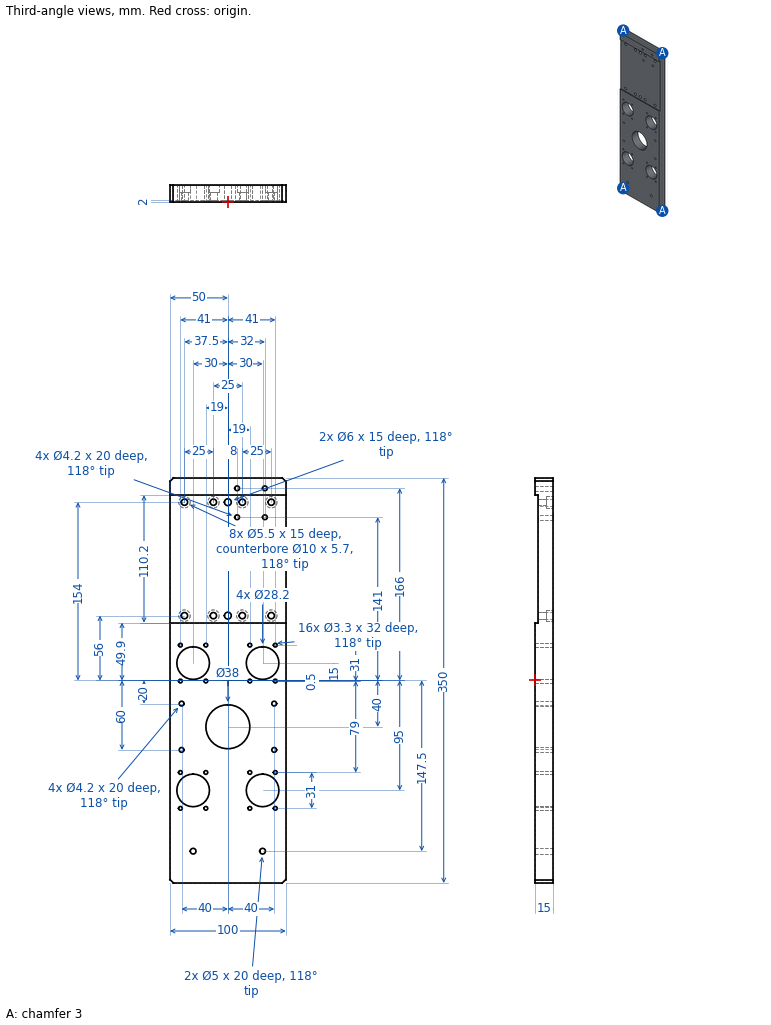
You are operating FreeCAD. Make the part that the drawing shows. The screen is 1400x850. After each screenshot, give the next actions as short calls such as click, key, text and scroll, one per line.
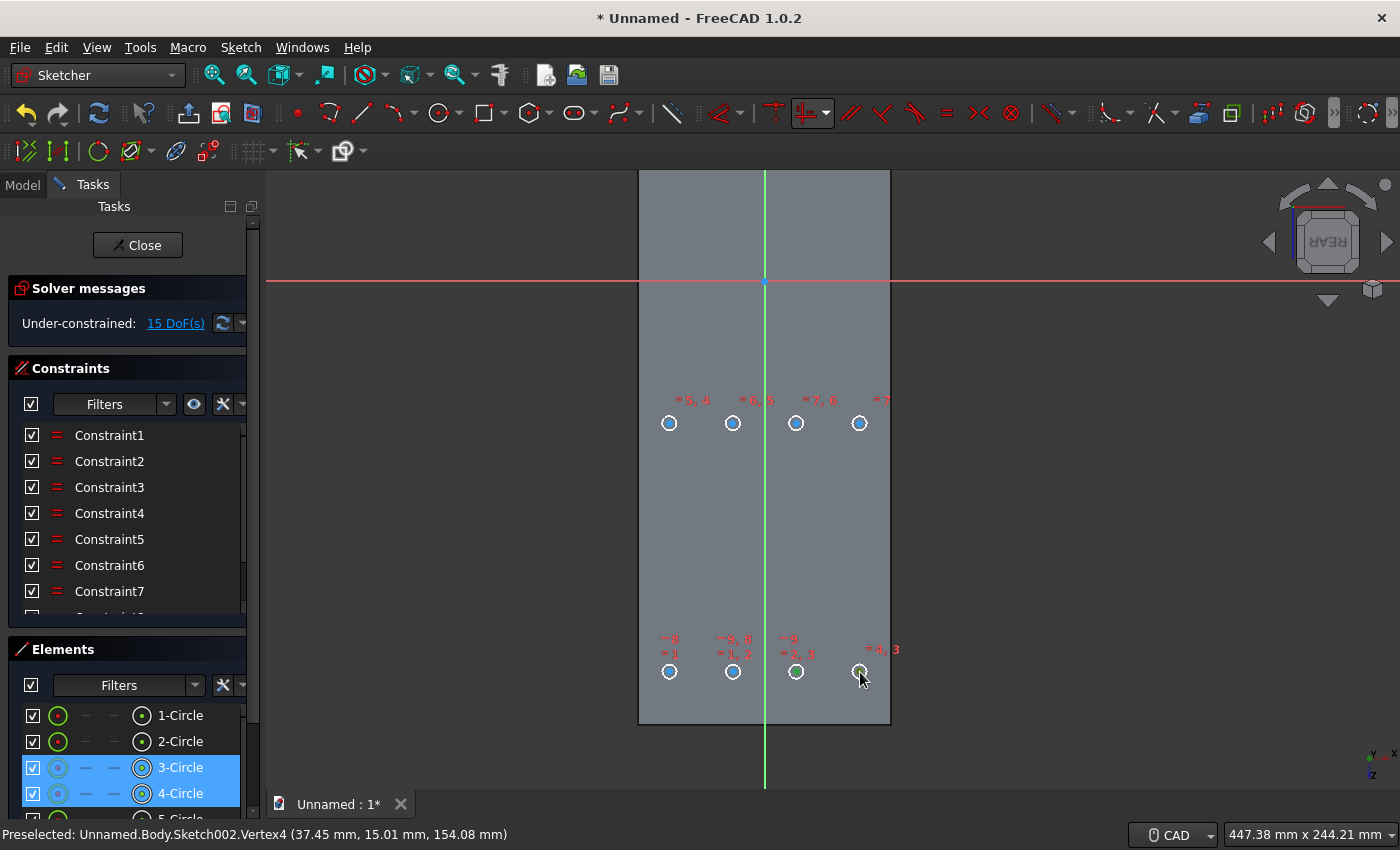
key(h)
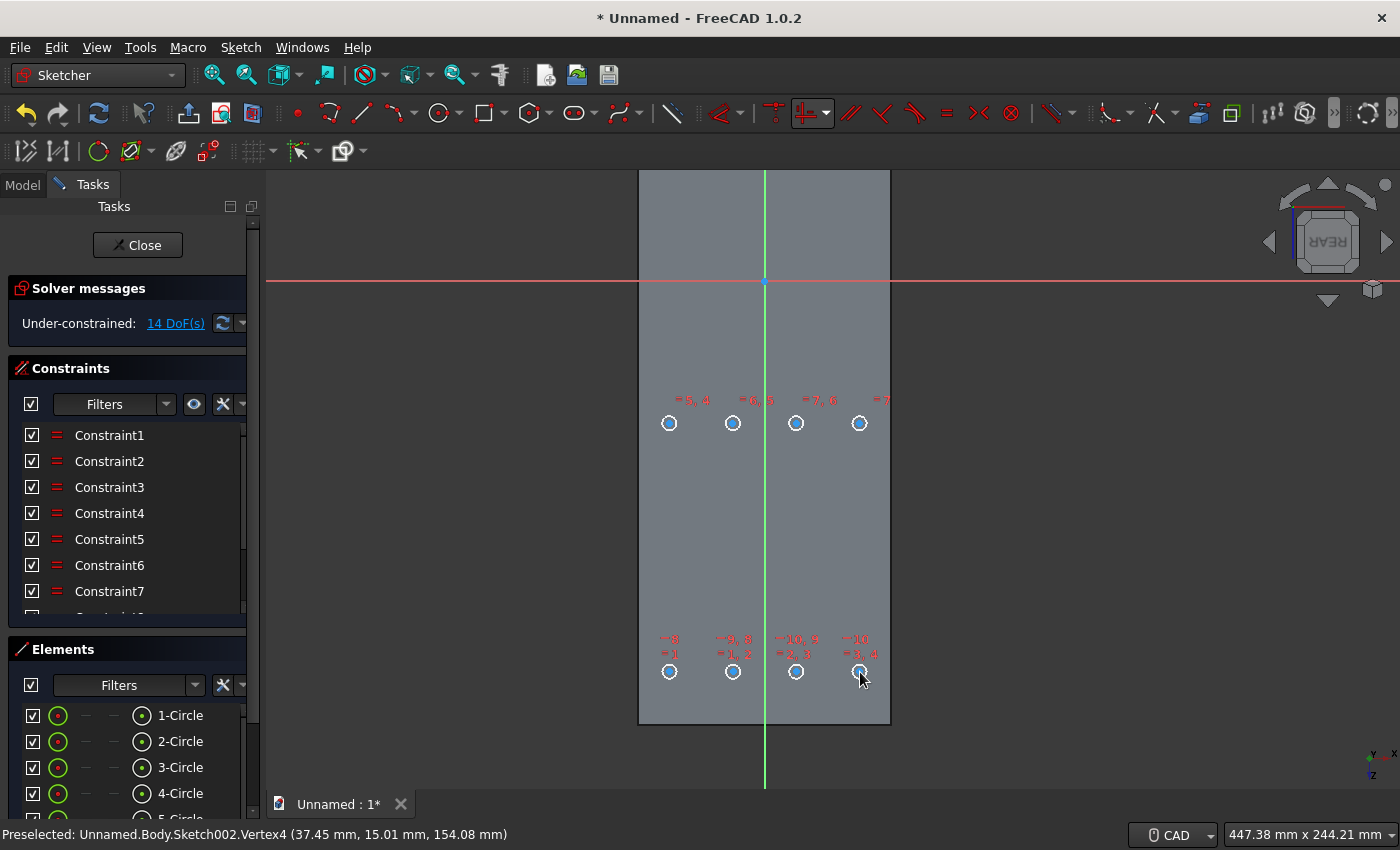
click(669, 672)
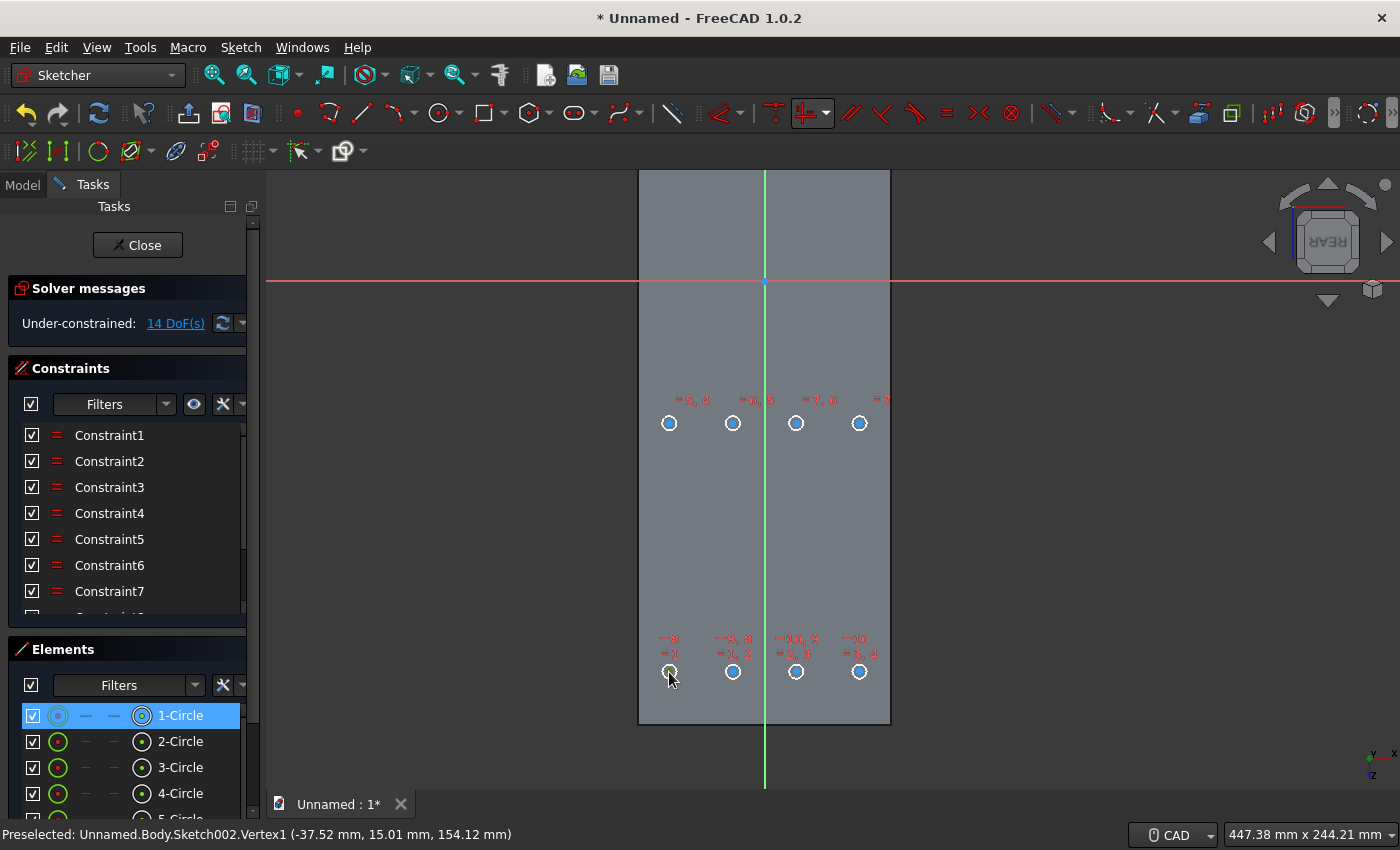
click(669, 423)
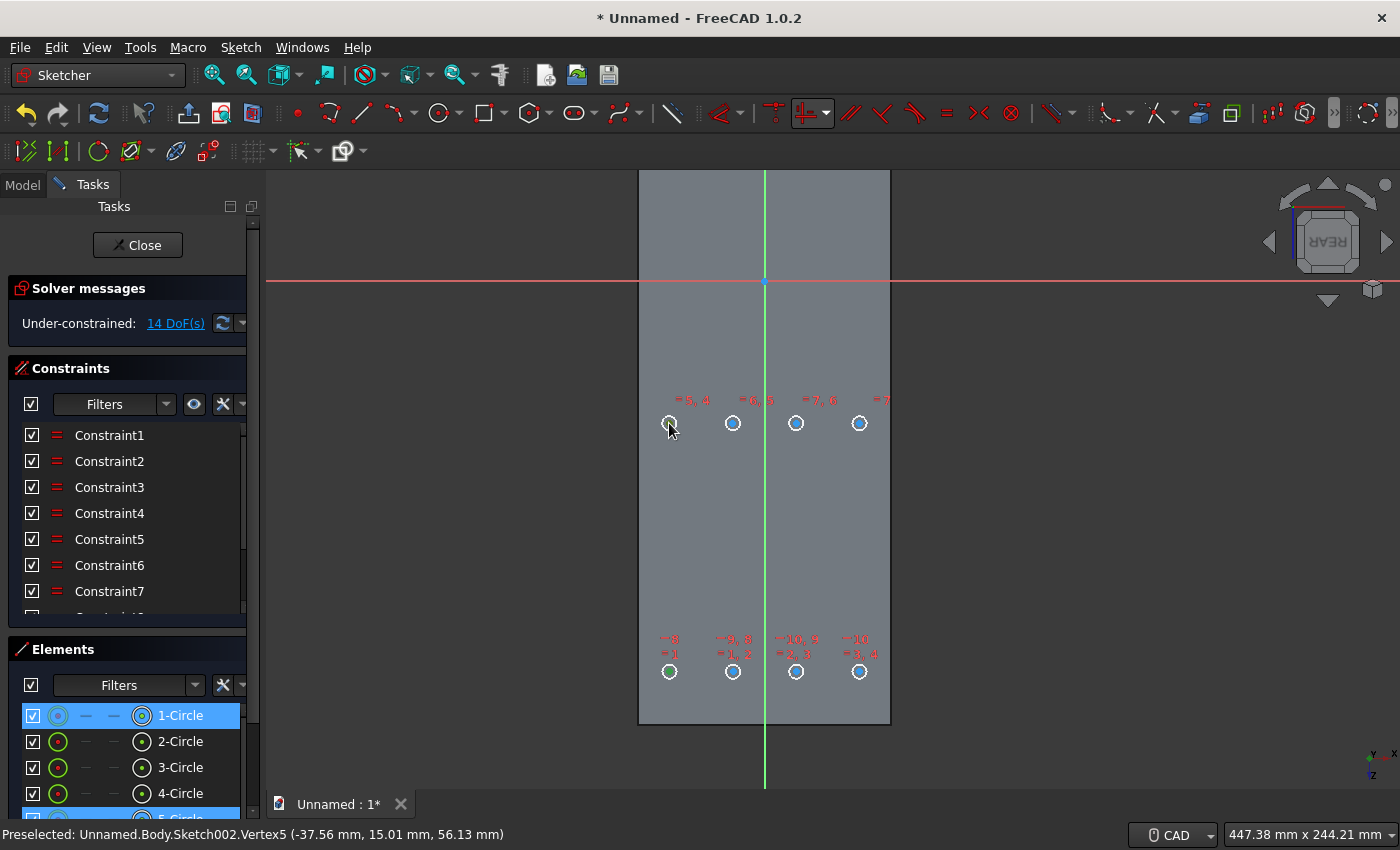
key(v)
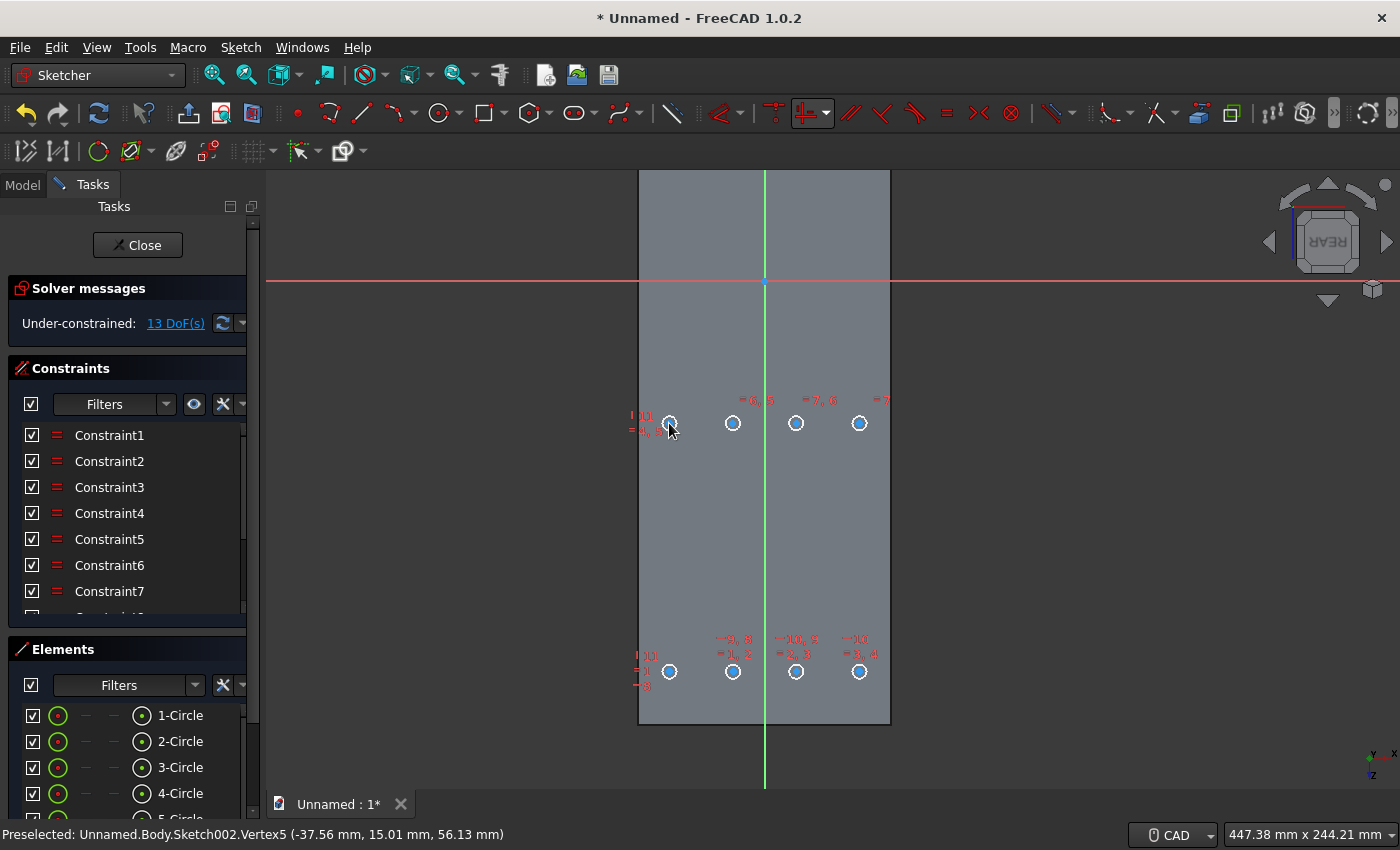
click(733, 672)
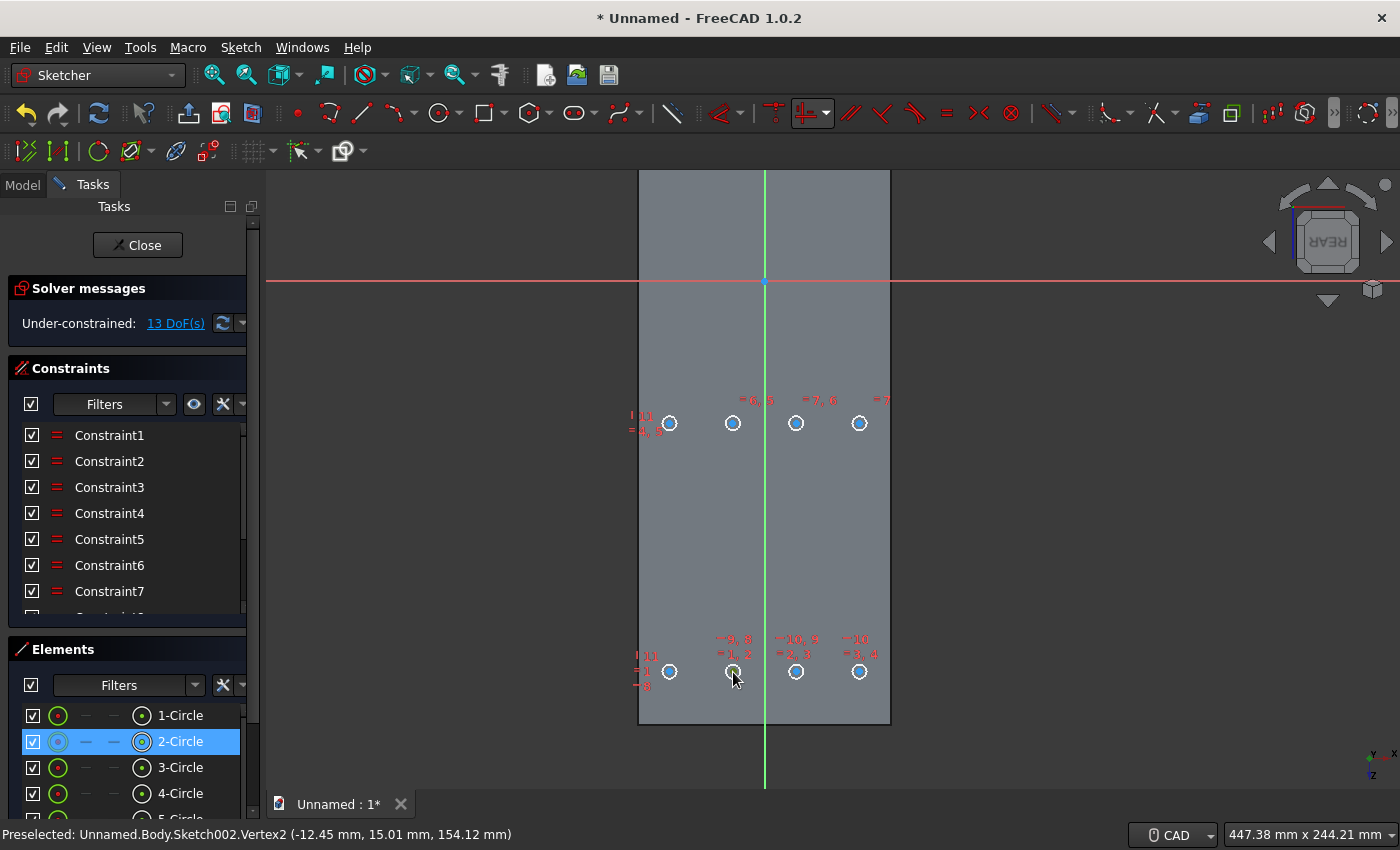
click(733, 423)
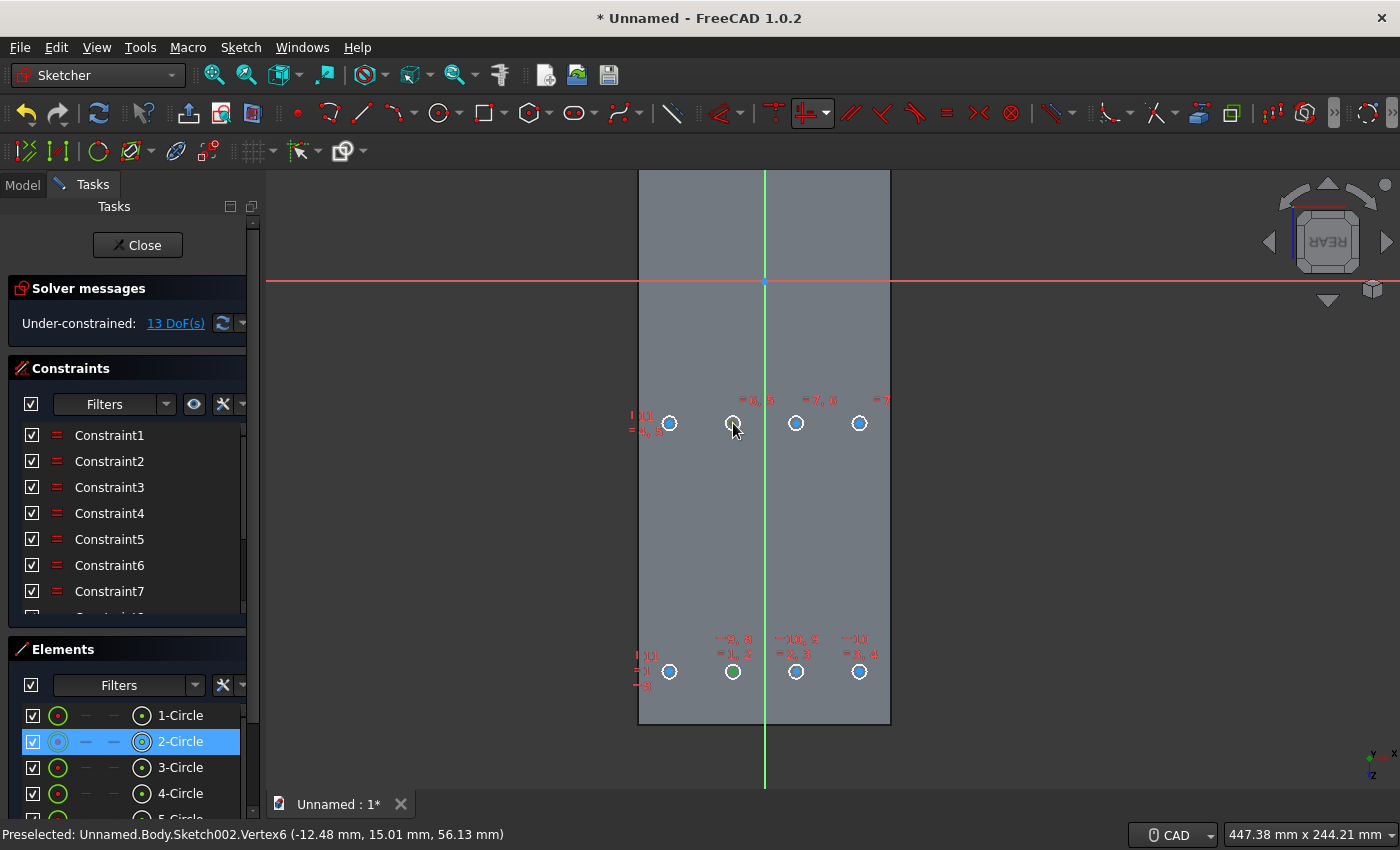
key(v)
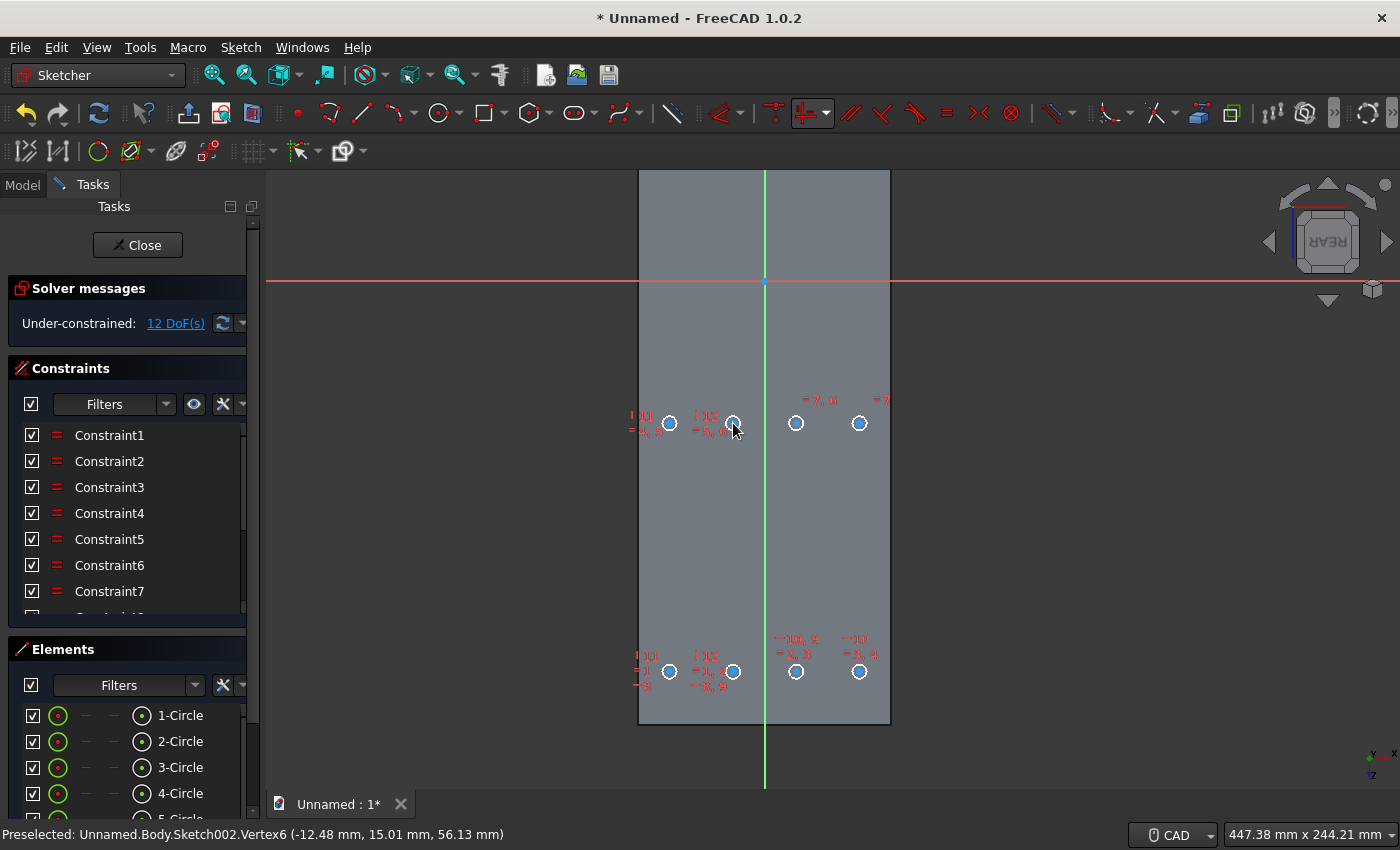
click(669, 423)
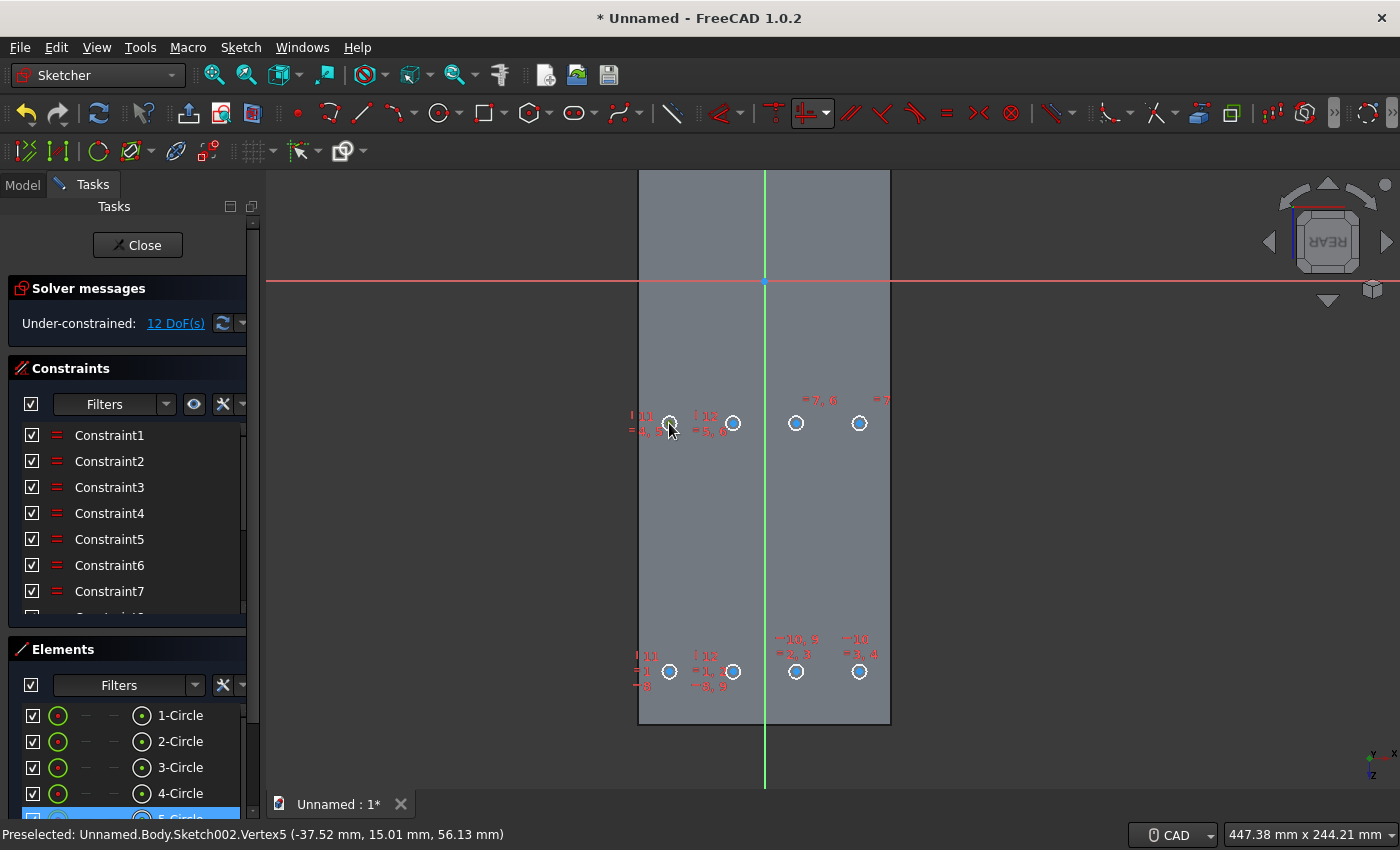
click(733, 423)